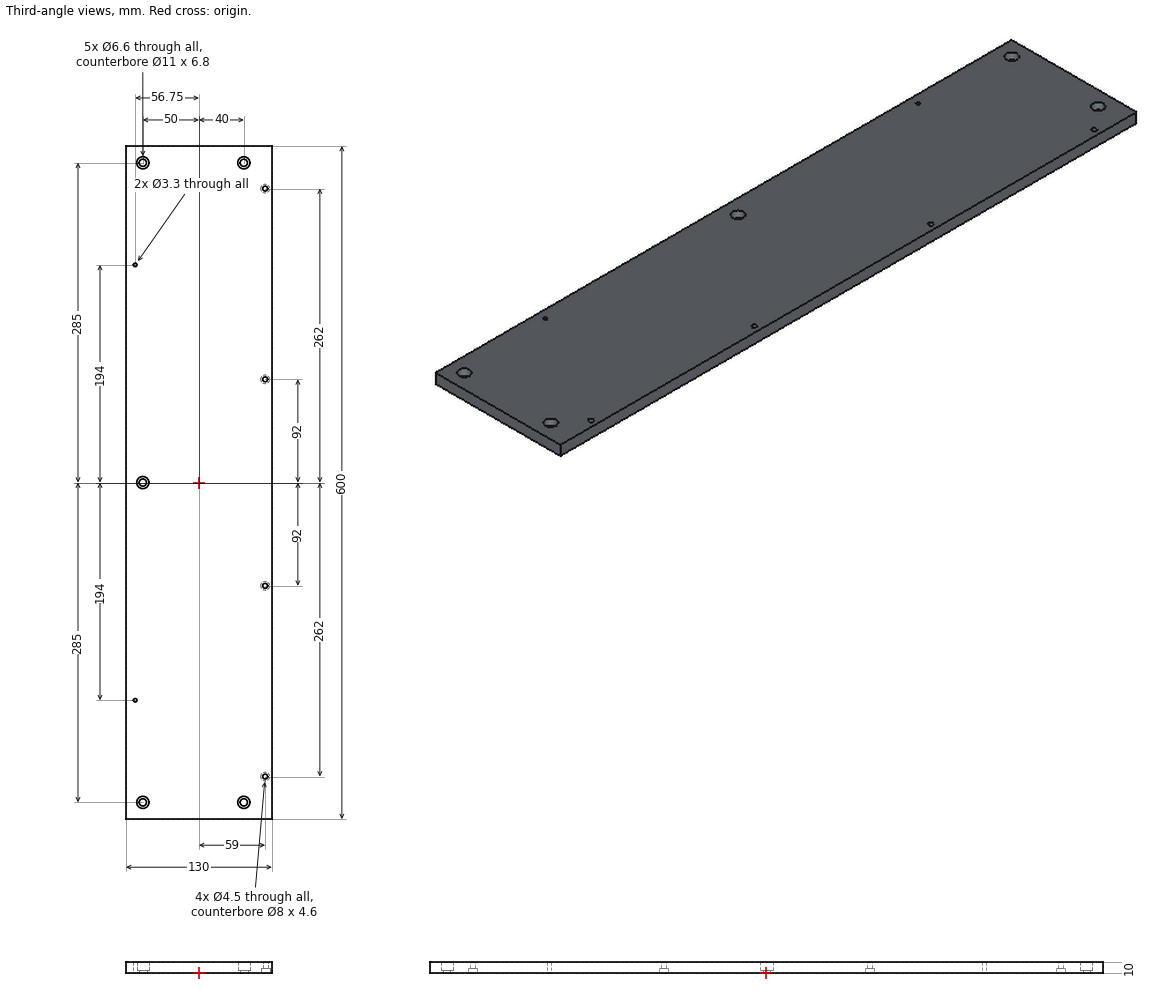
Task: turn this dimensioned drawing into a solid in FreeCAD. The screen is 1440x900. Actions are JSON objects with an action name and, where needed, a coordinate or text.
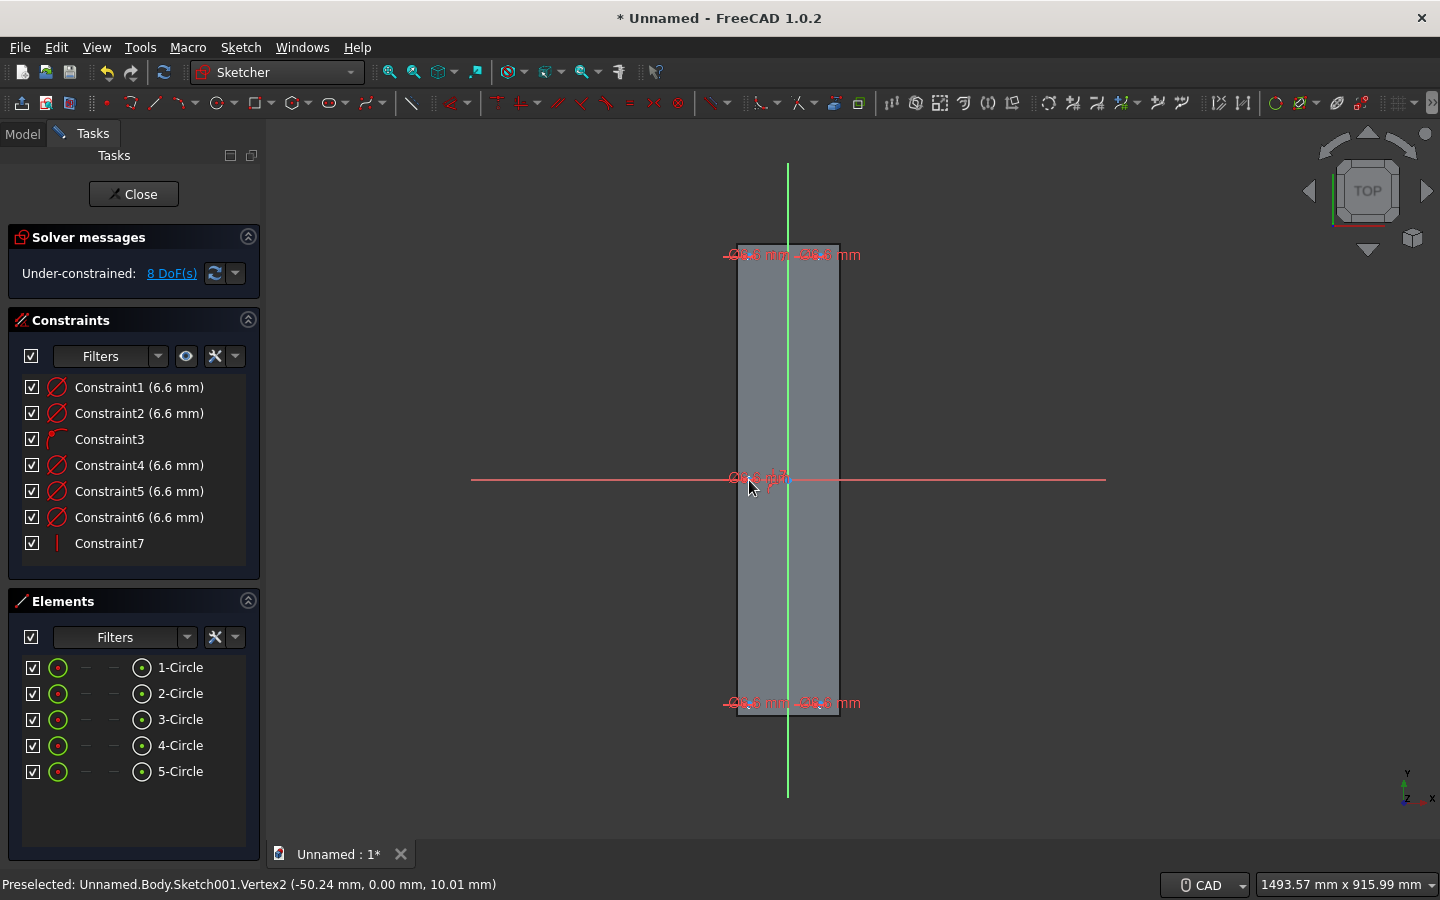
{"action": "left_click", "coordinate": [749, 480]}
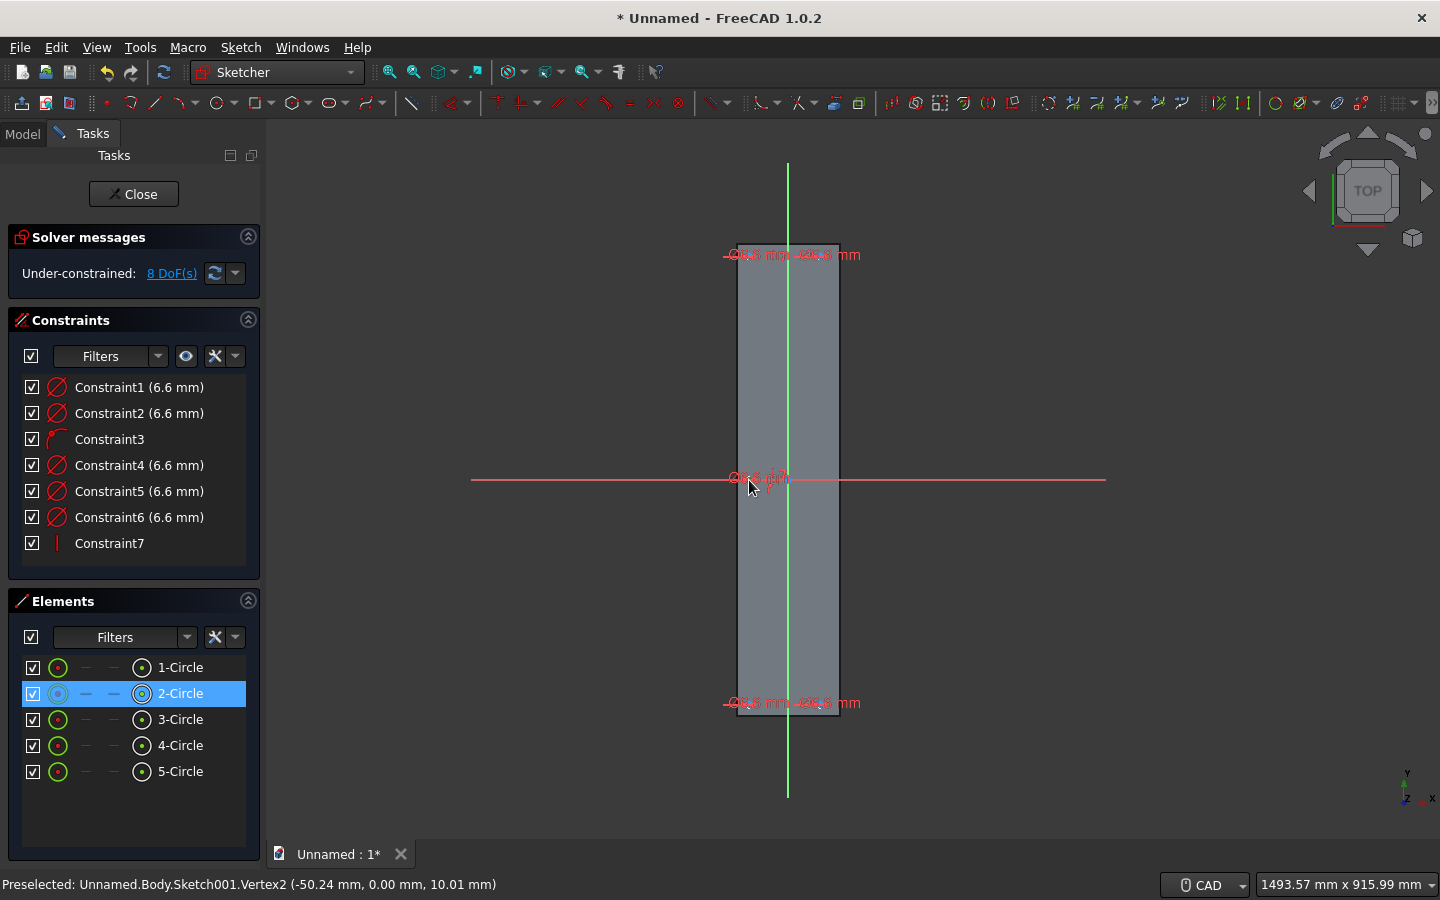
{"action": "left_click", "coordinate": [749, 705]}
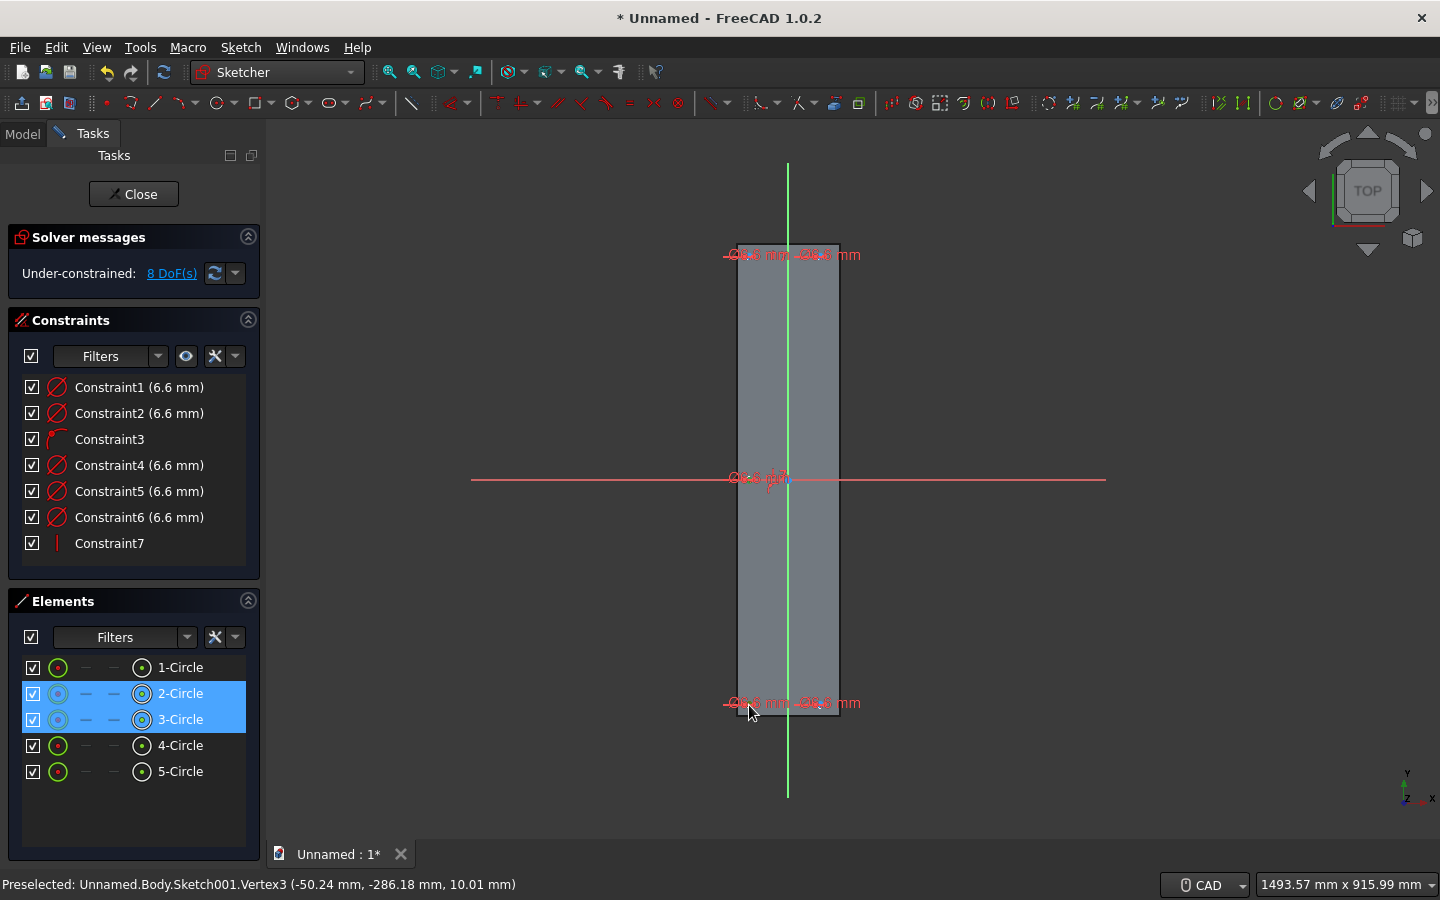
{"action": "key", "text": "v"}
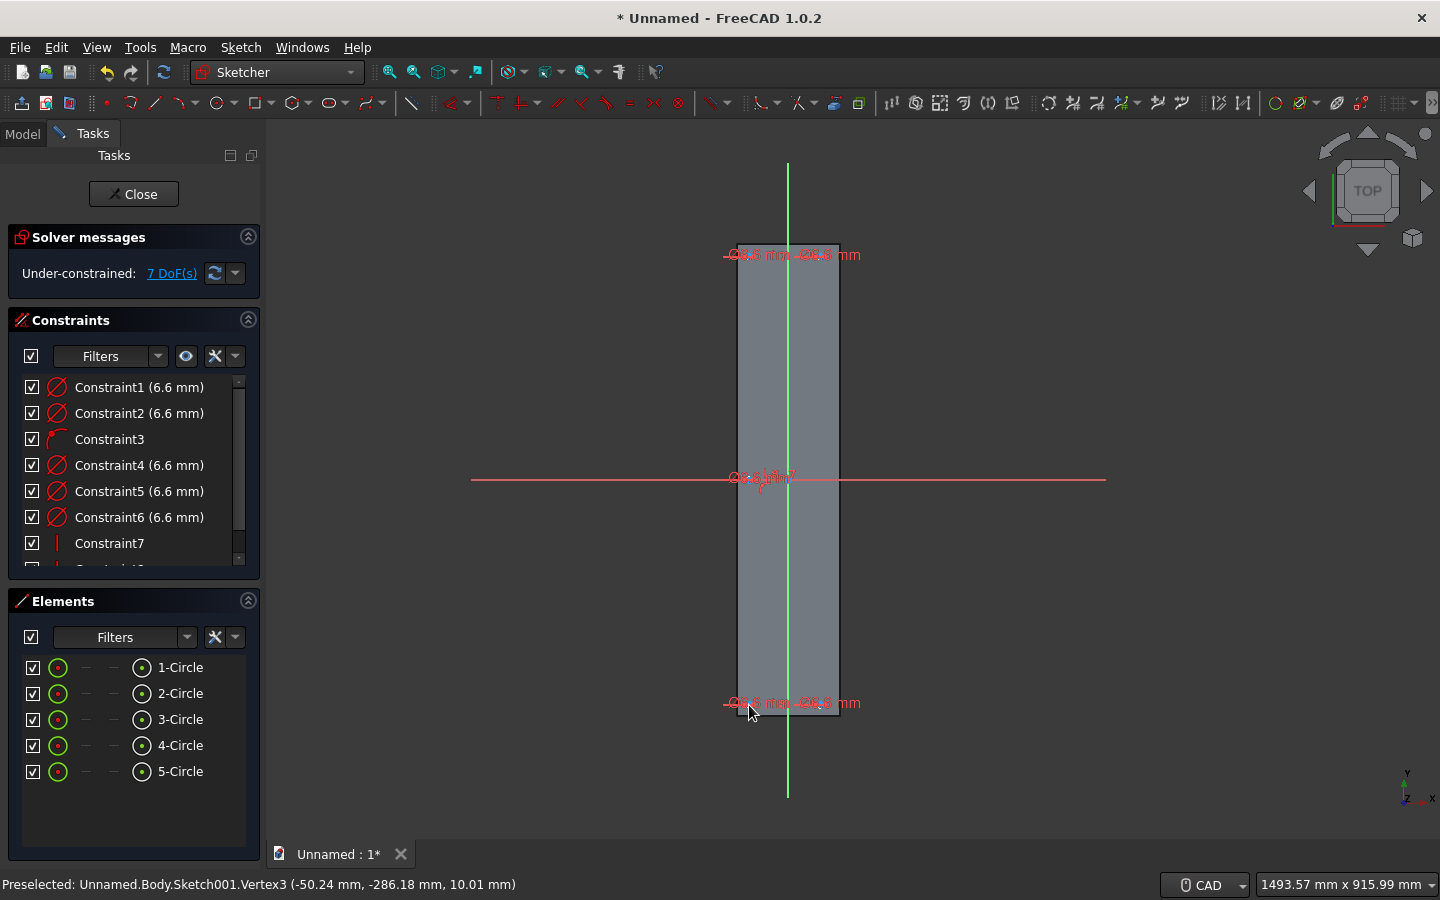
{"action": "left_click", "coordinate": [749, 257]}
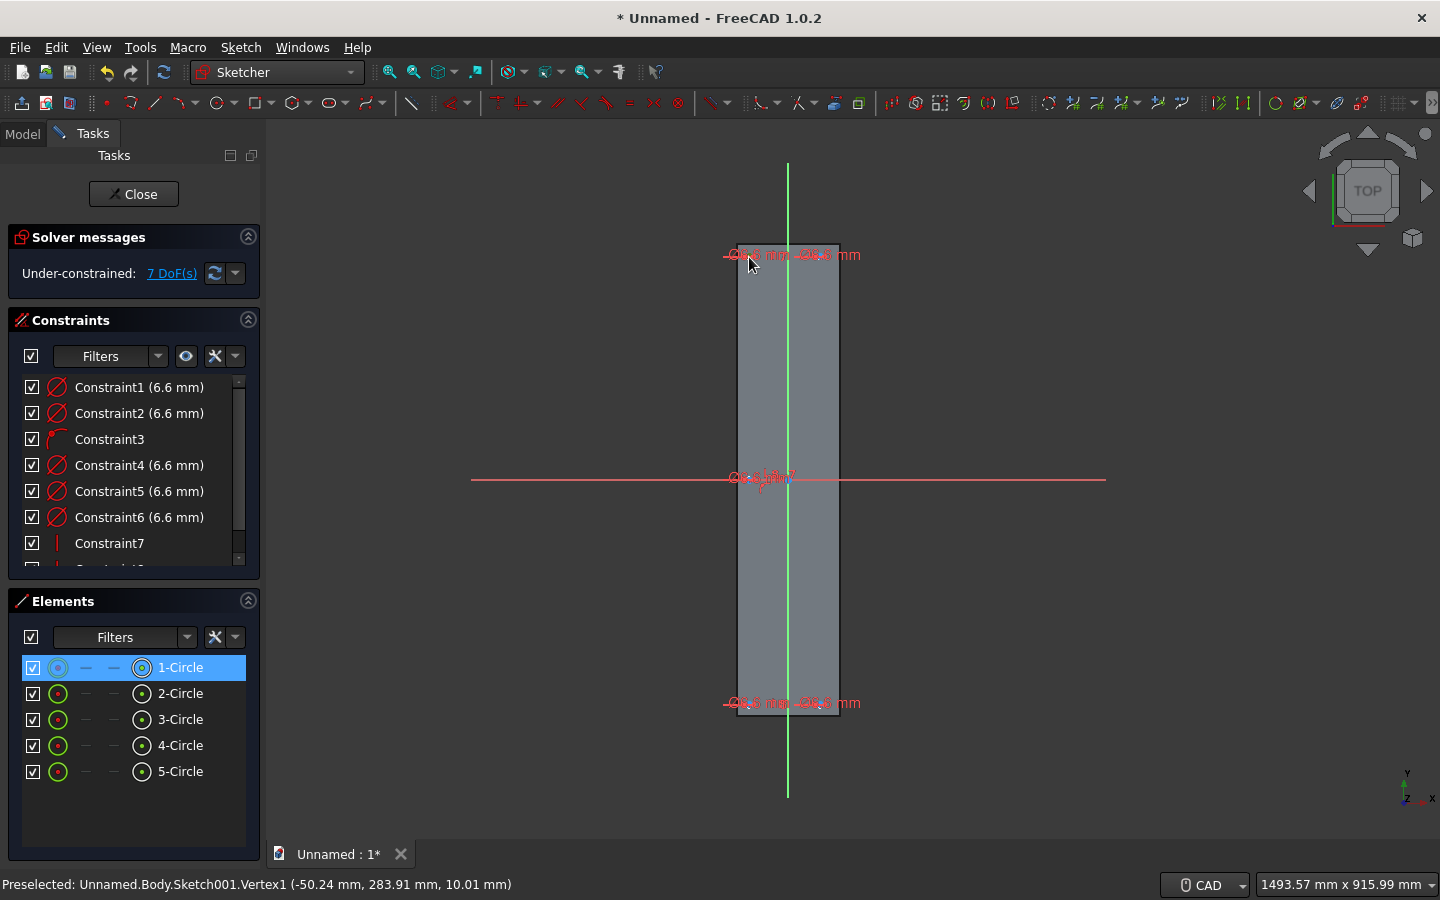
{"action": "left_click", "coordinate": [820, 257]}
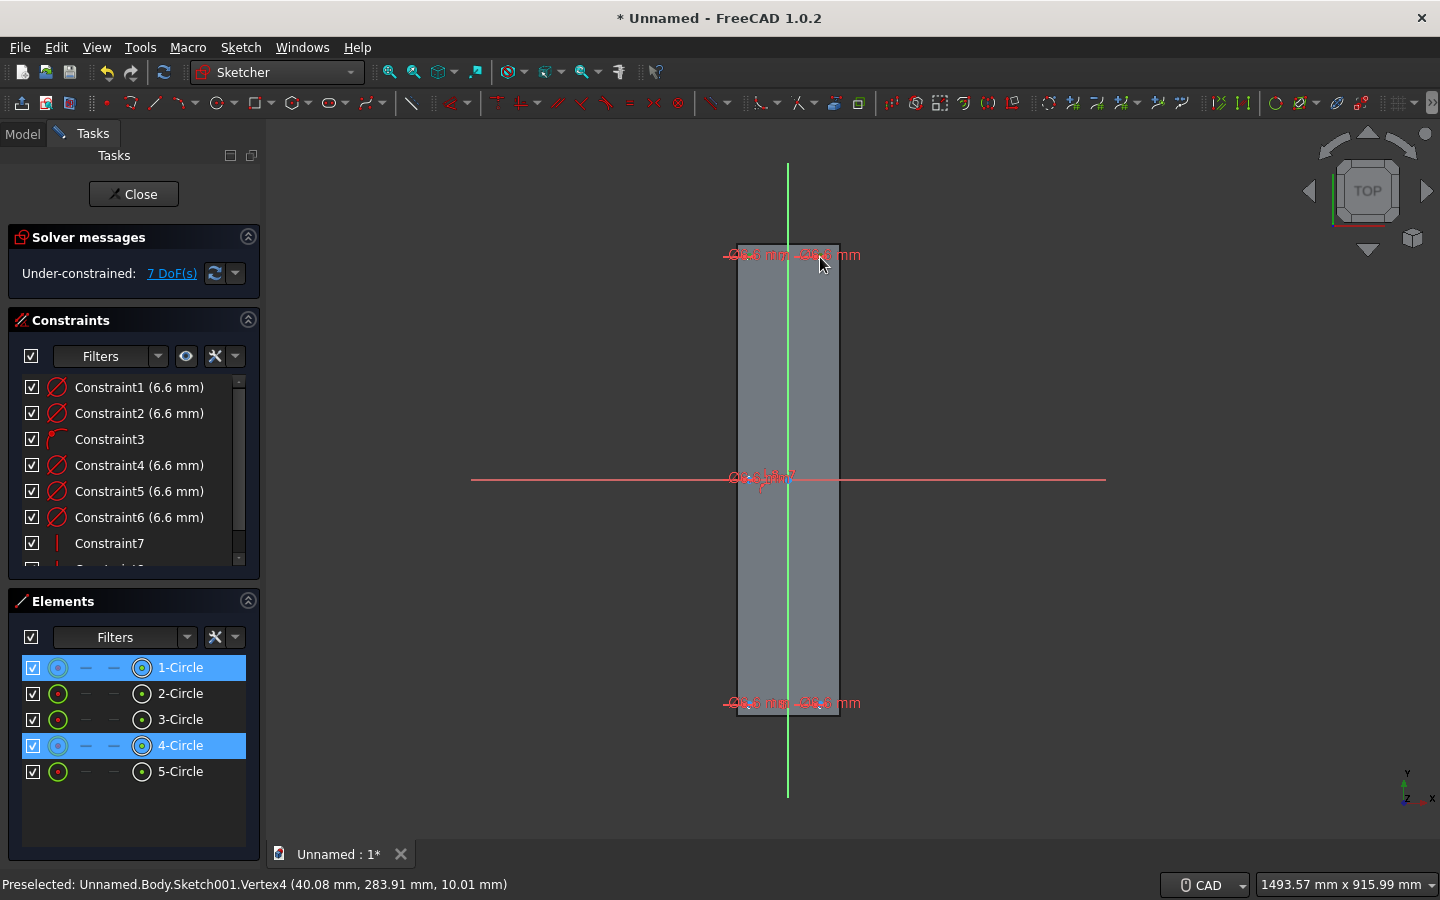
{"action": "key", "text": "h"}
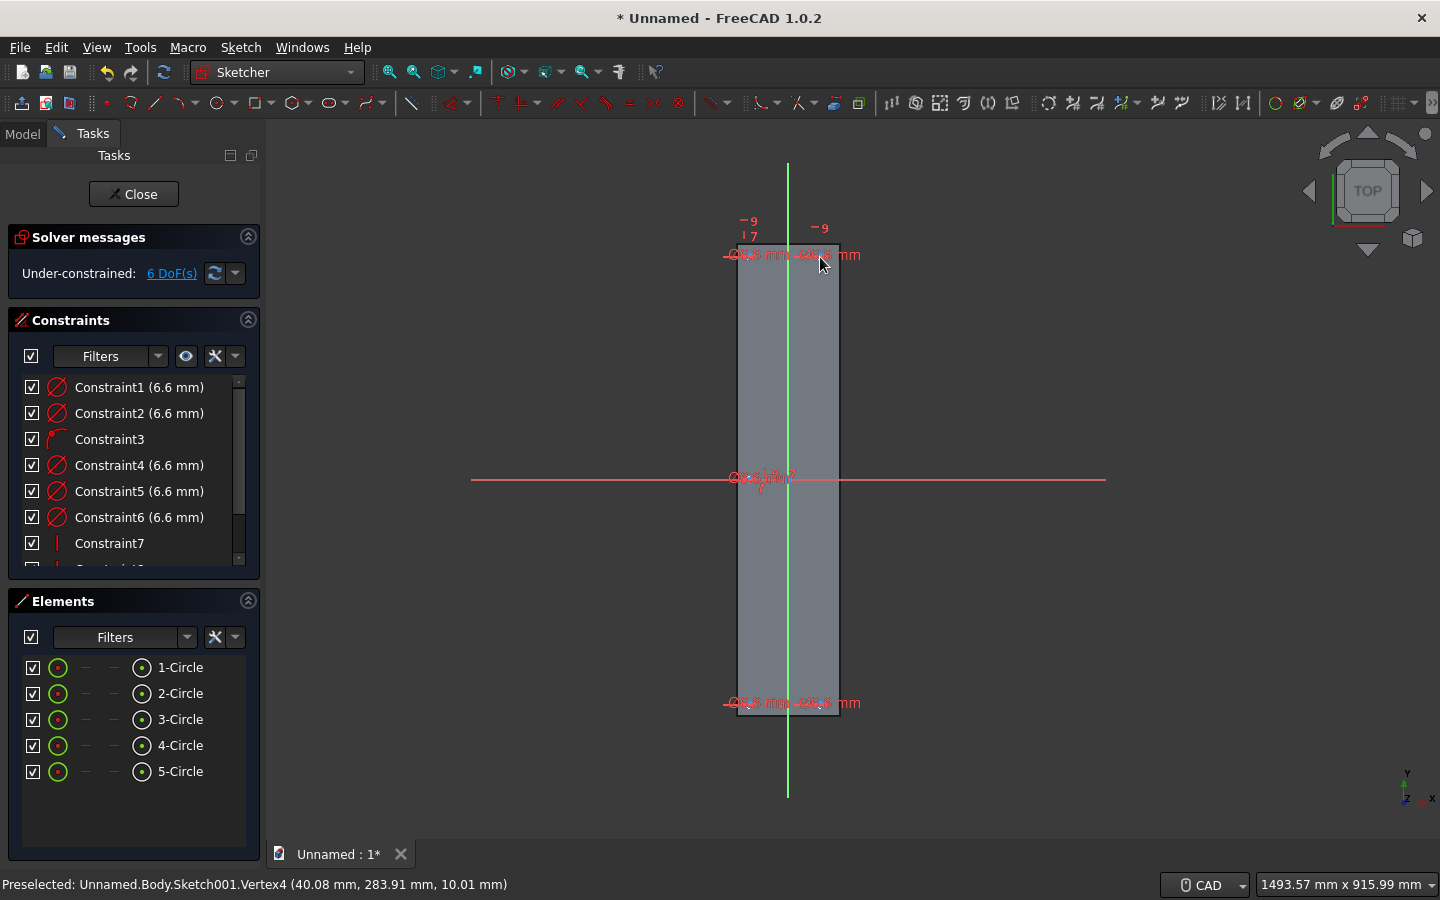
{"action": "left_click", "coordinate": [820, 257]}